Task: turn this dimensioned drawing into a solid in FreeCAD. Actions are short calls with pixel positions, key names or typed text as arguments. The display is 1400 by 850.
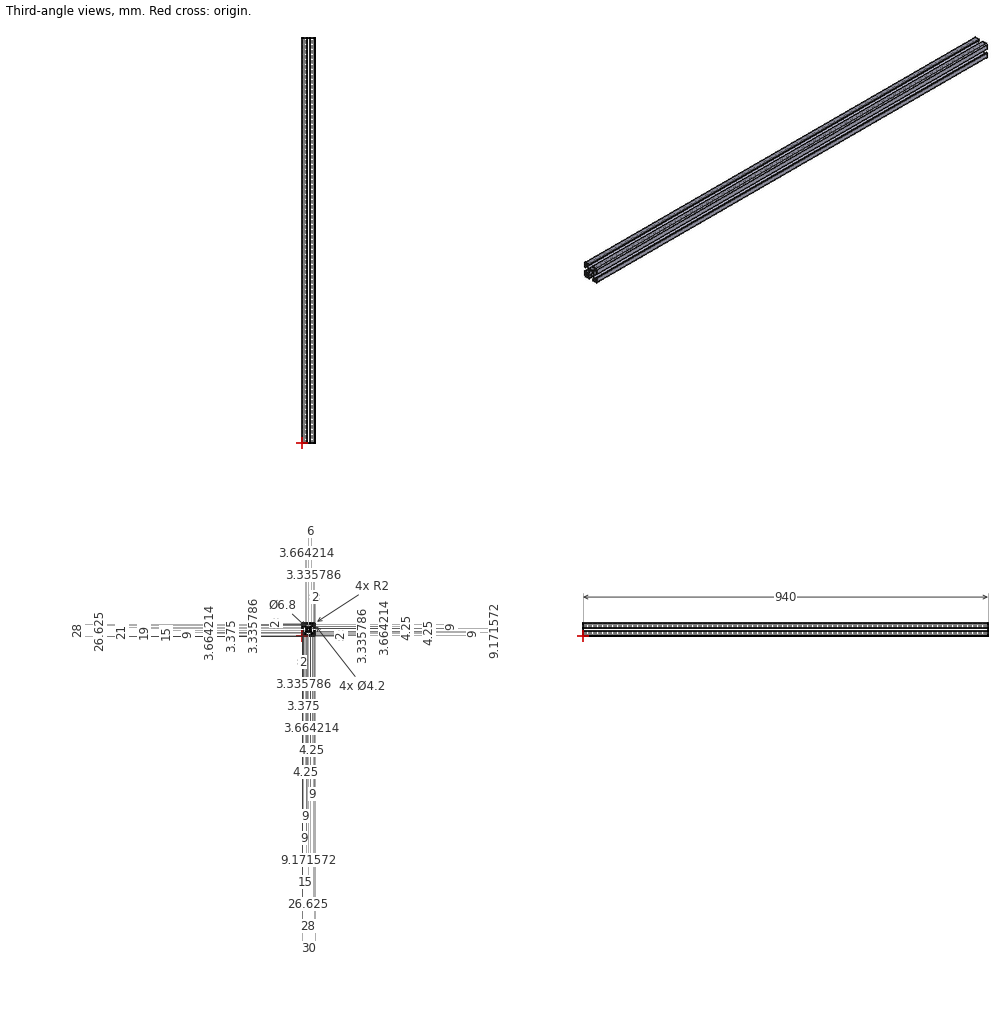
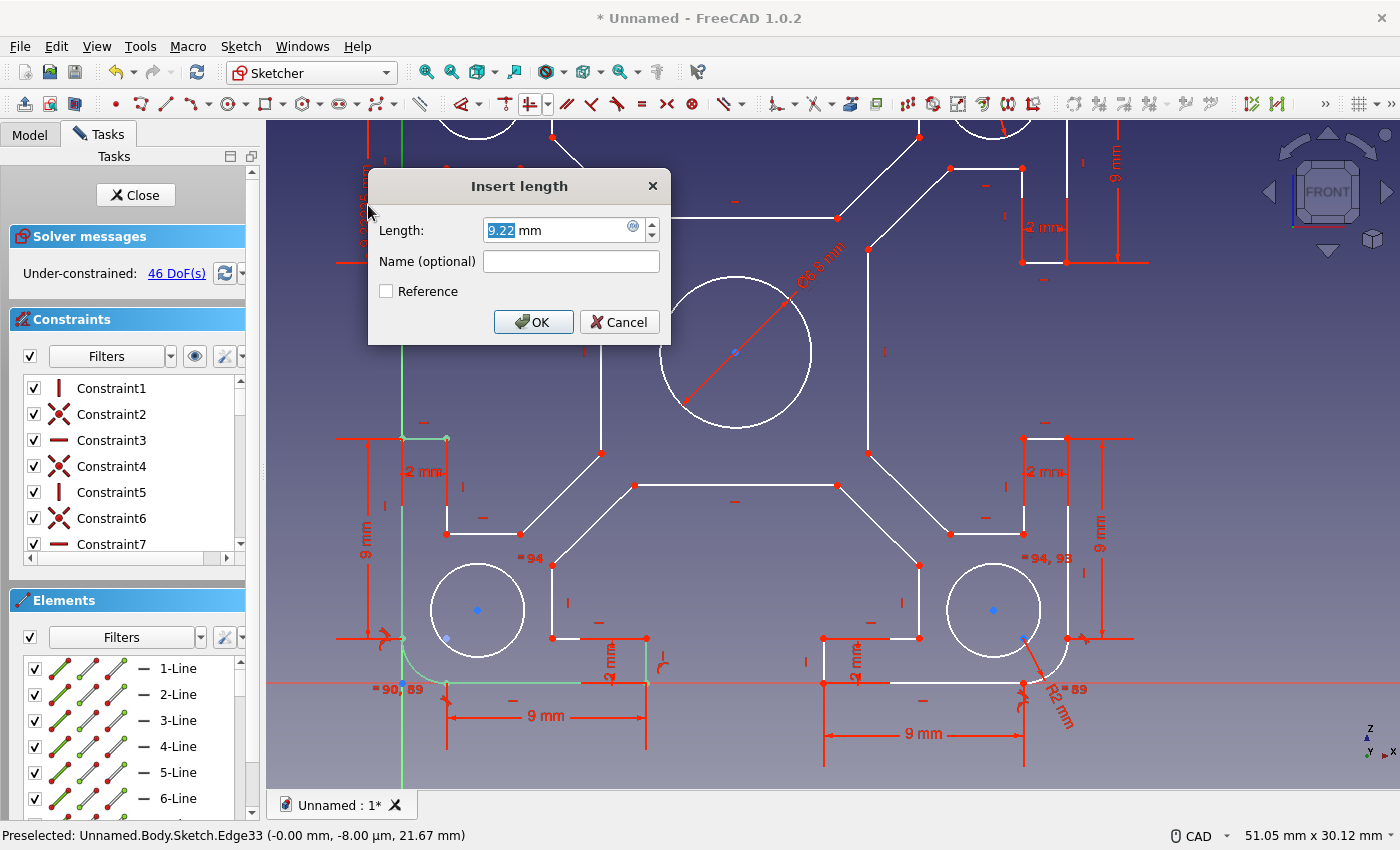
text(9)
key(Return)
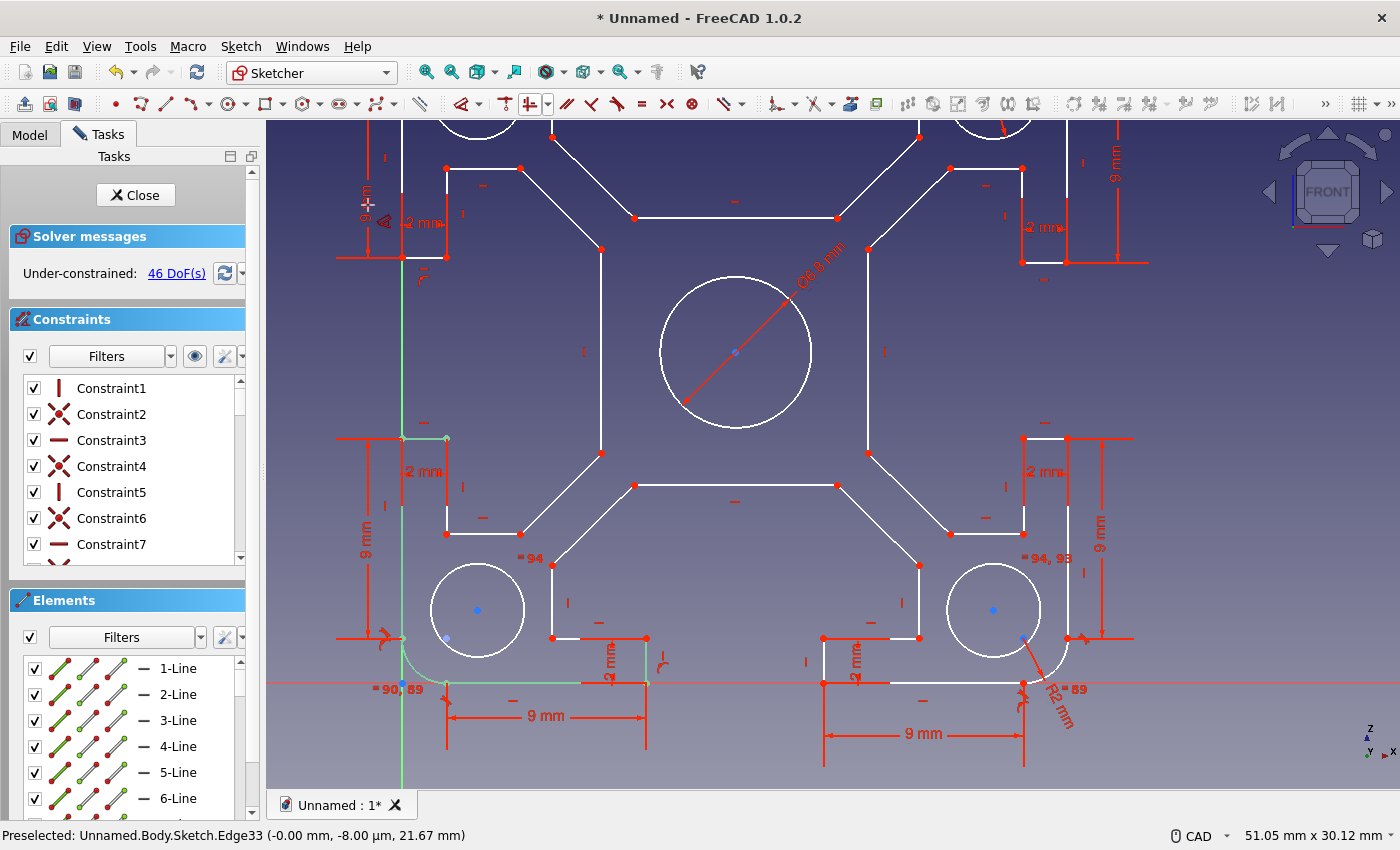
scroll(824, 667, down, 2)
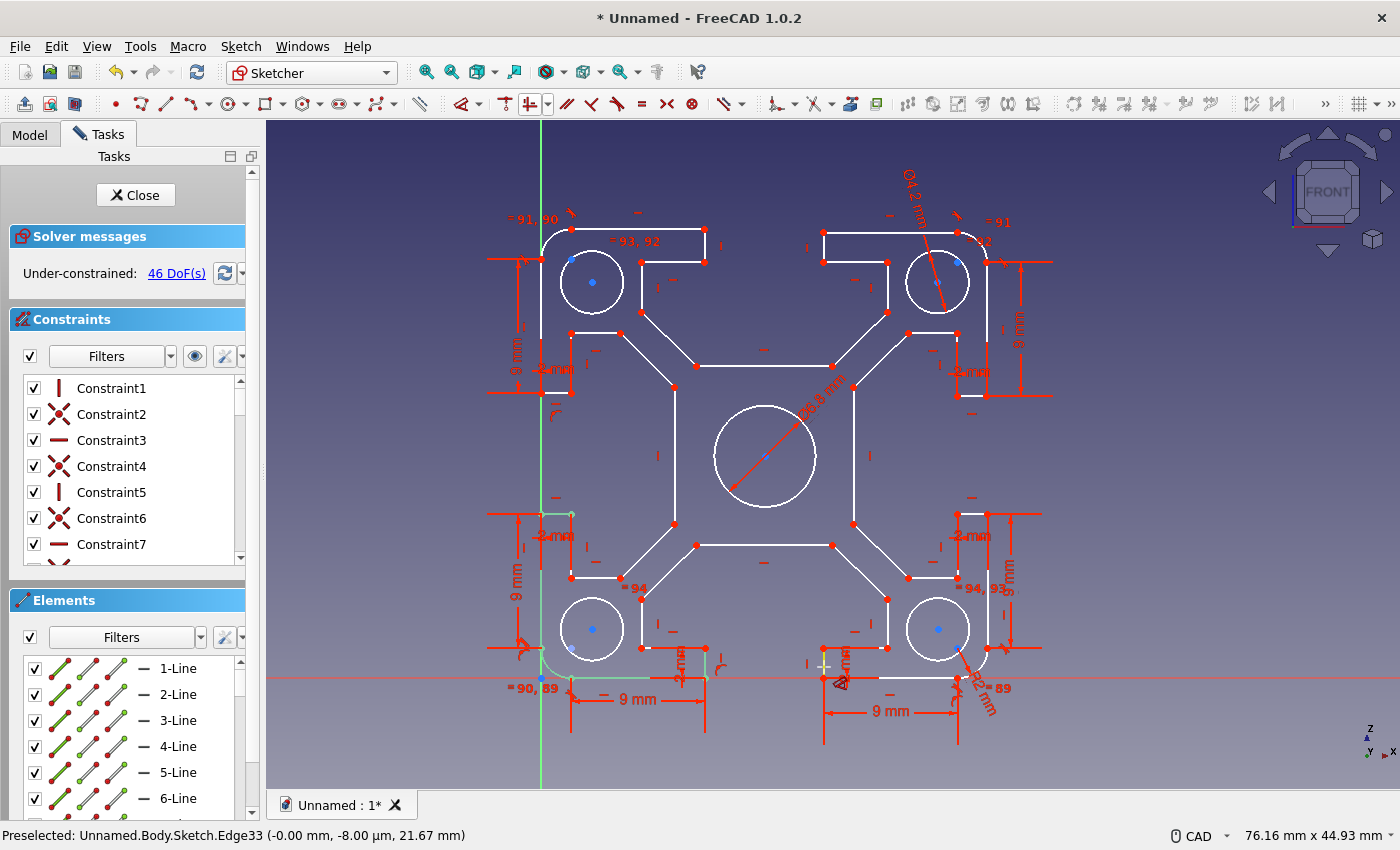
click(611, 229)
click(638, 195)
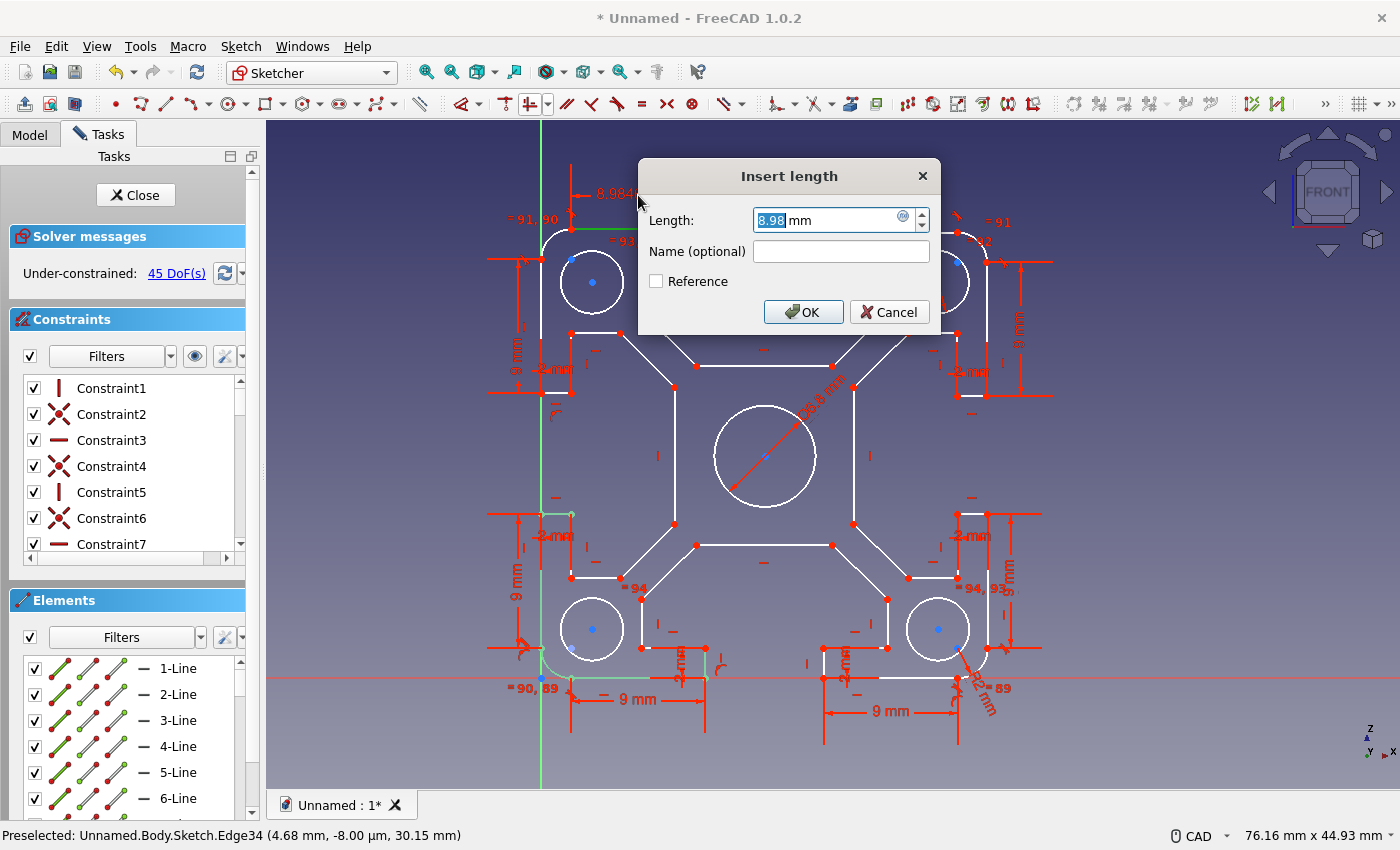
text(9)
key(Return)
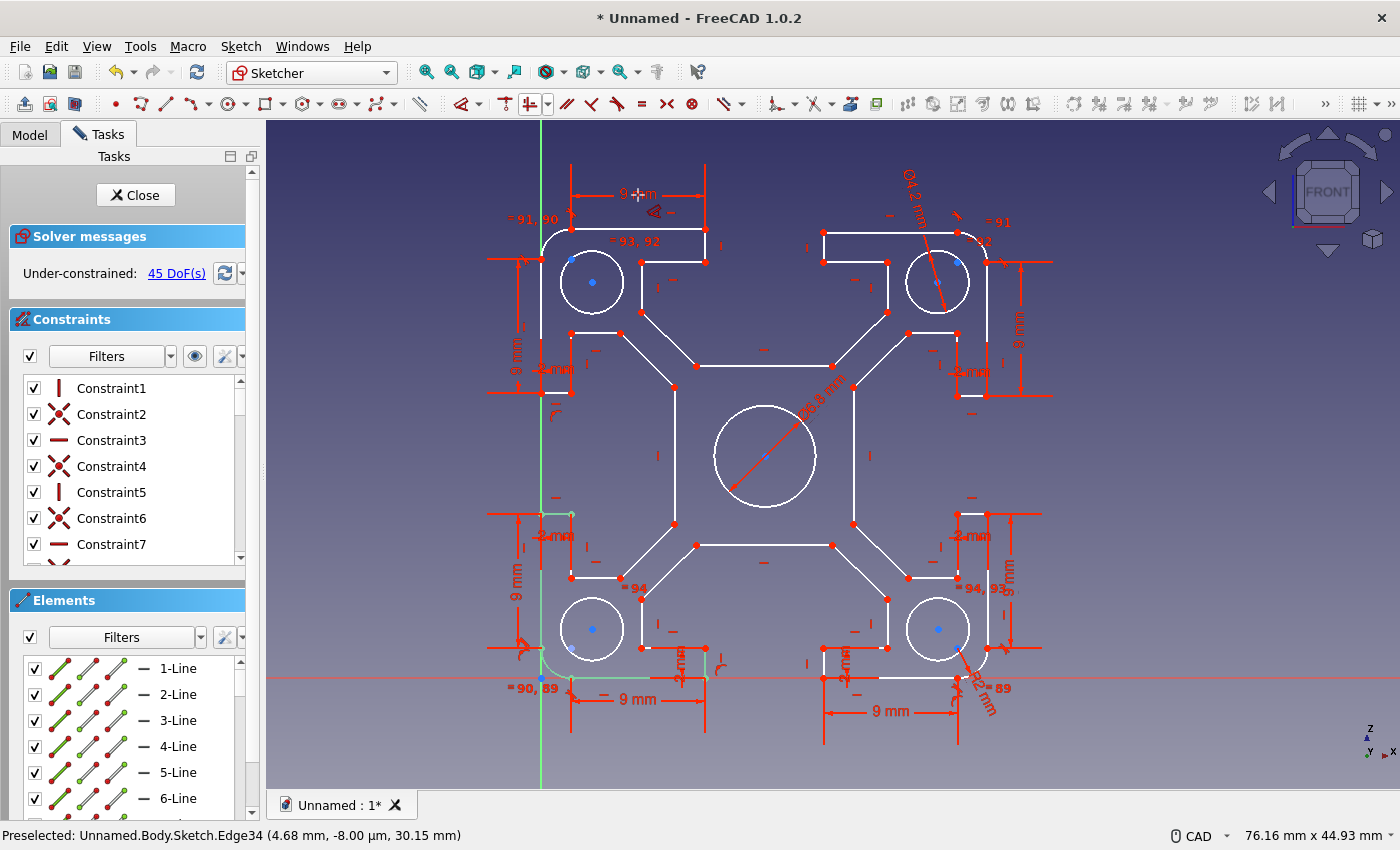
scroll(705, 239, up, 2)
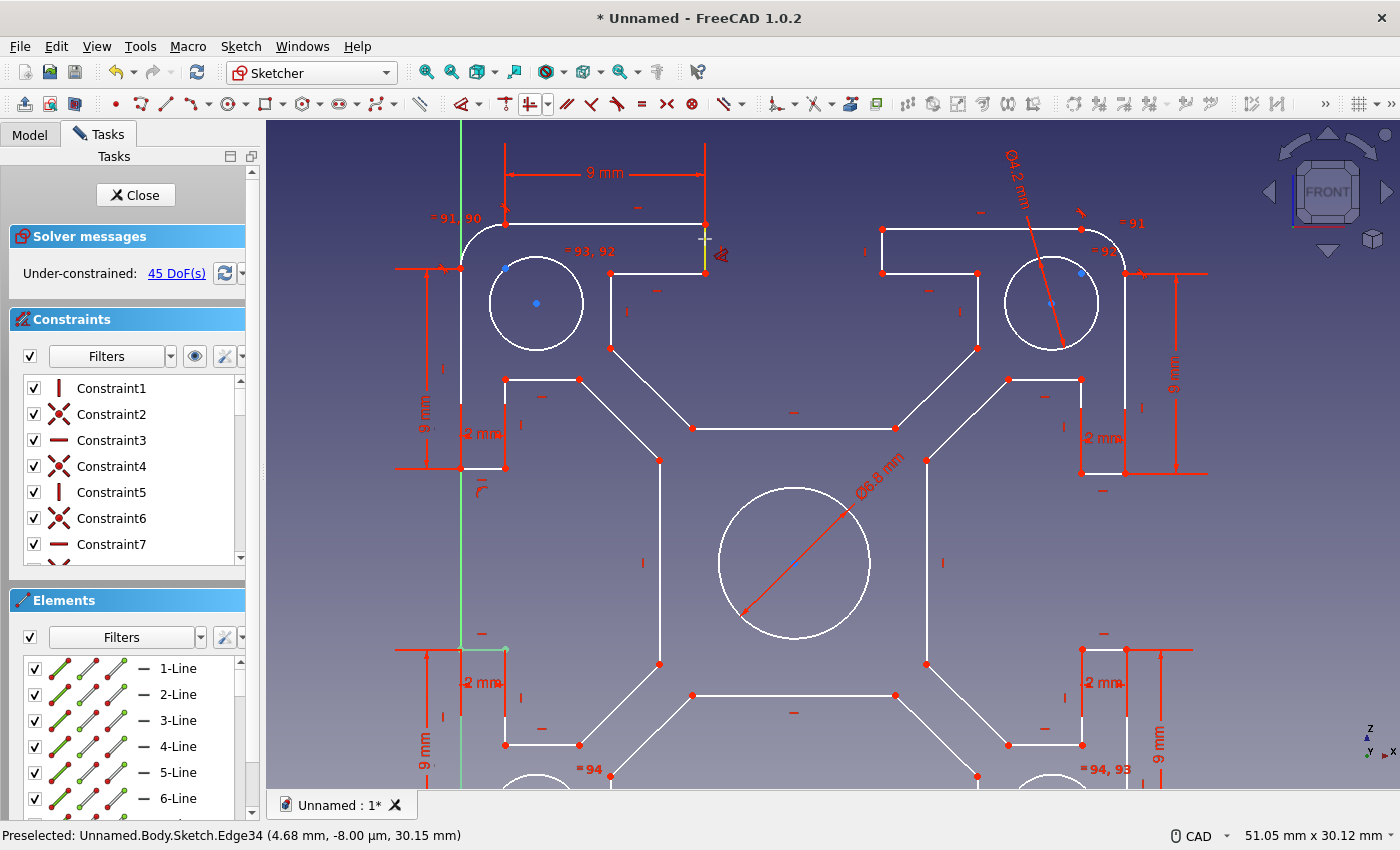
click(705, 239)
click(671, 249)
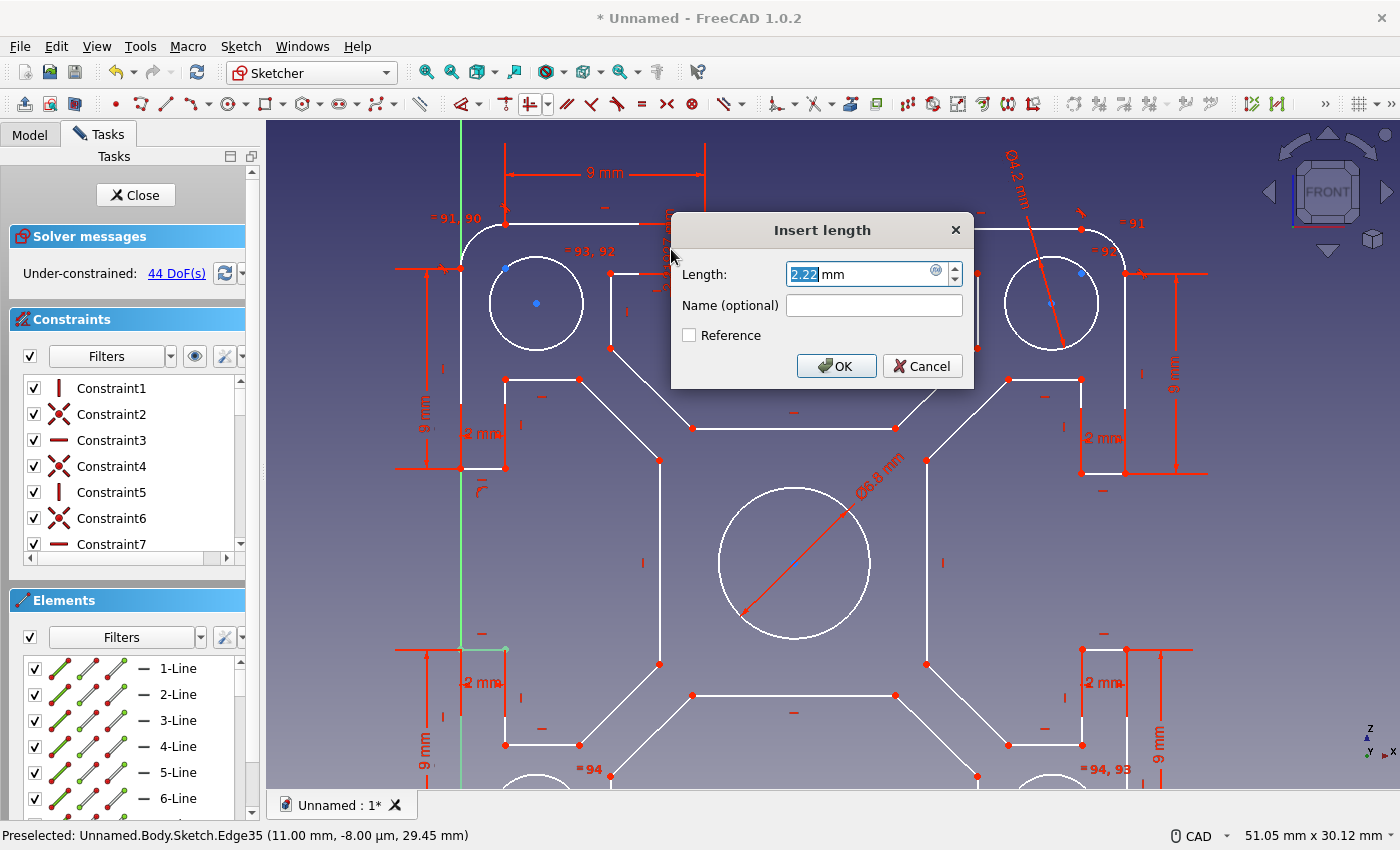
text(2)
key(Return)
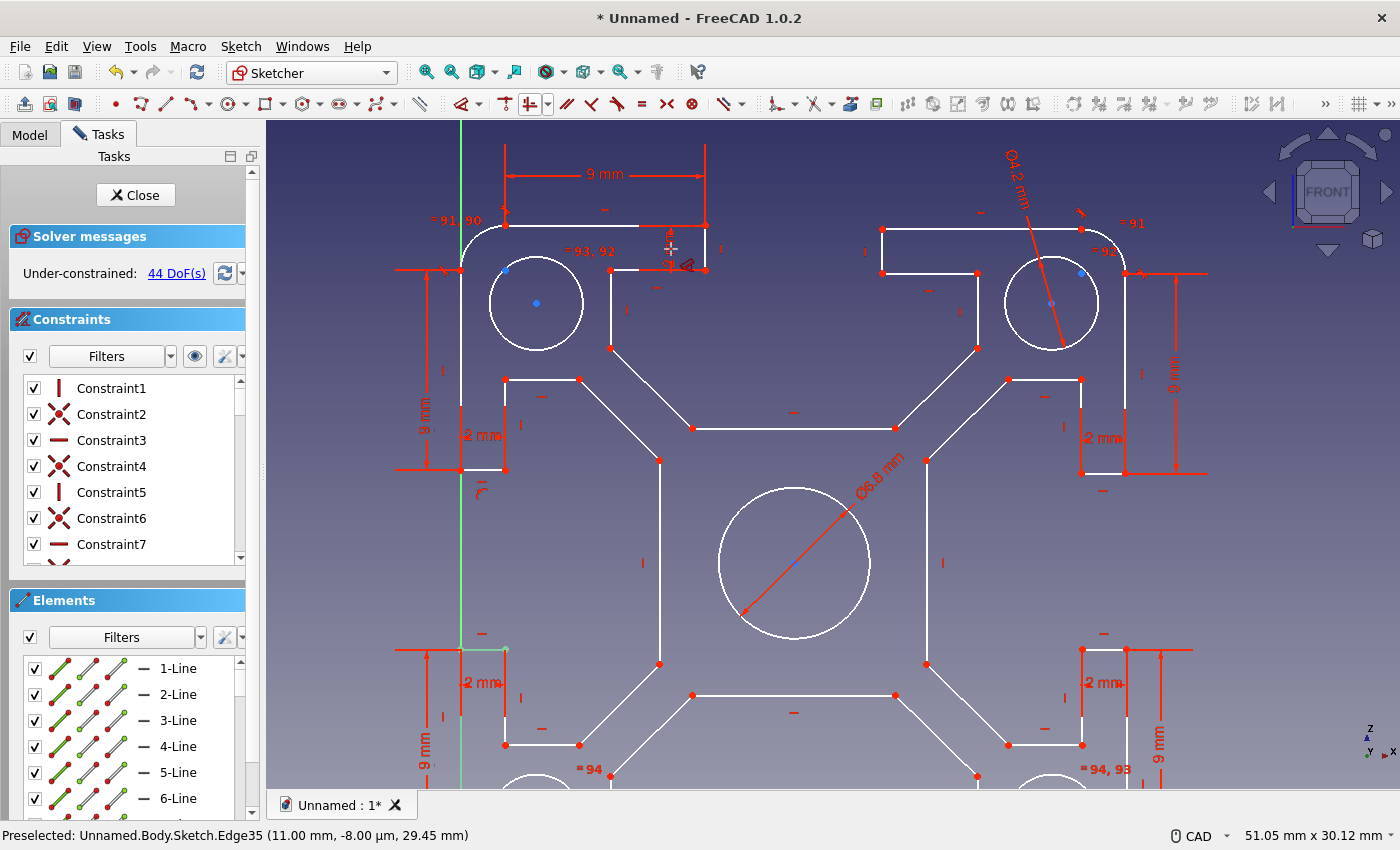
click(882, 260)
click(916, 252)